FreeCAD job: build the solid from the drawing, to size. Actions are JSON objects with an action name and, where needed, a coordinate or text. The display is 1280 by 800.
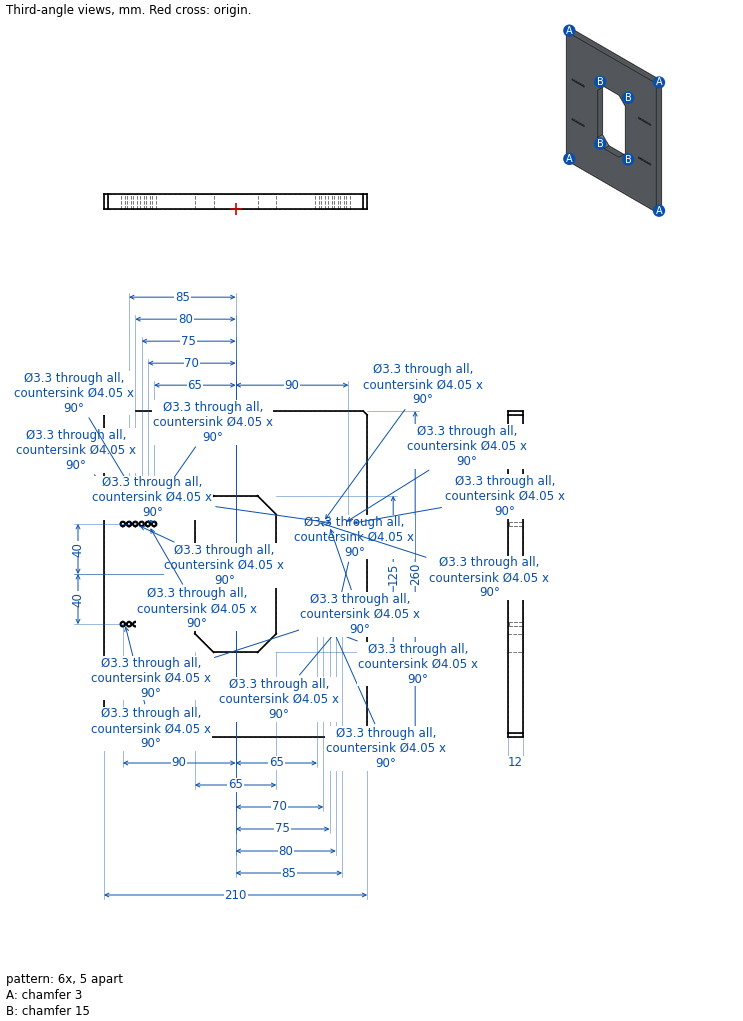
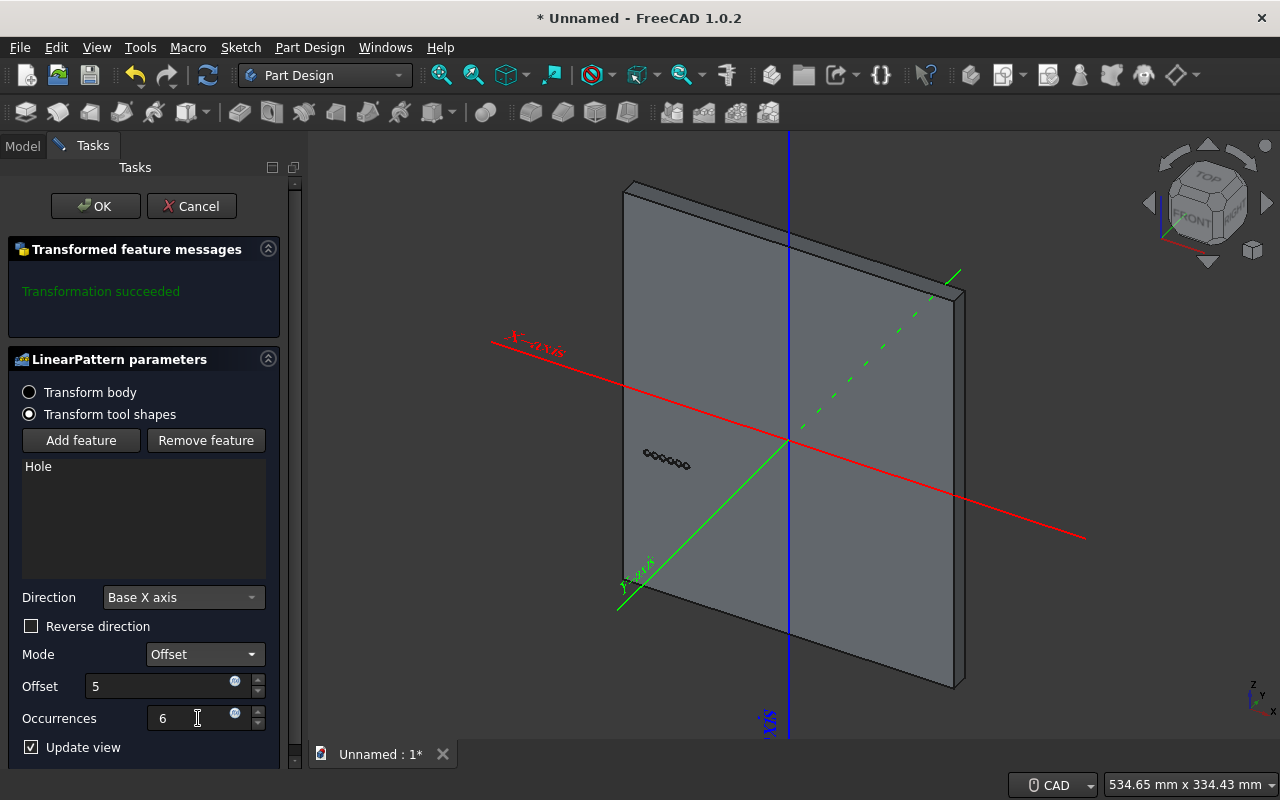
{"action": "left_click", "coordinate": [96, 206]}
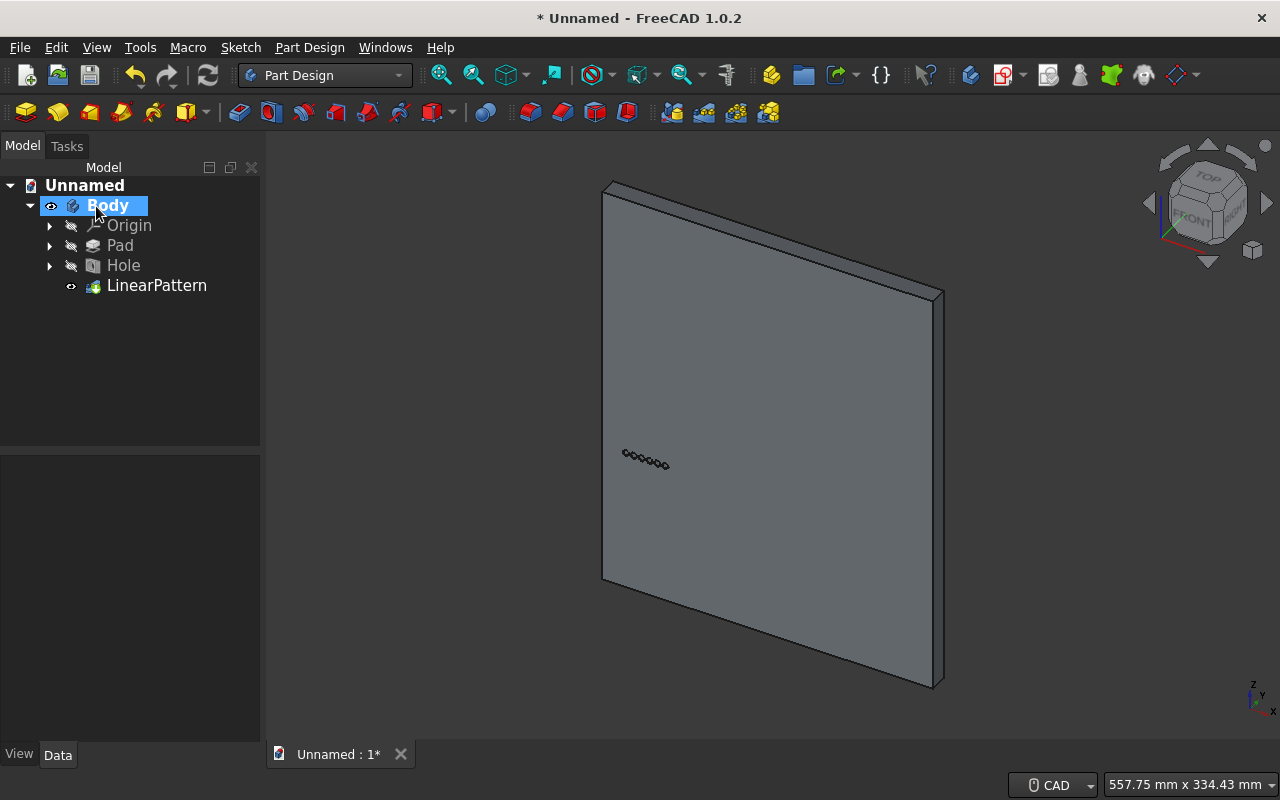
{"action": "left_click", "coordinate": [116, 266]}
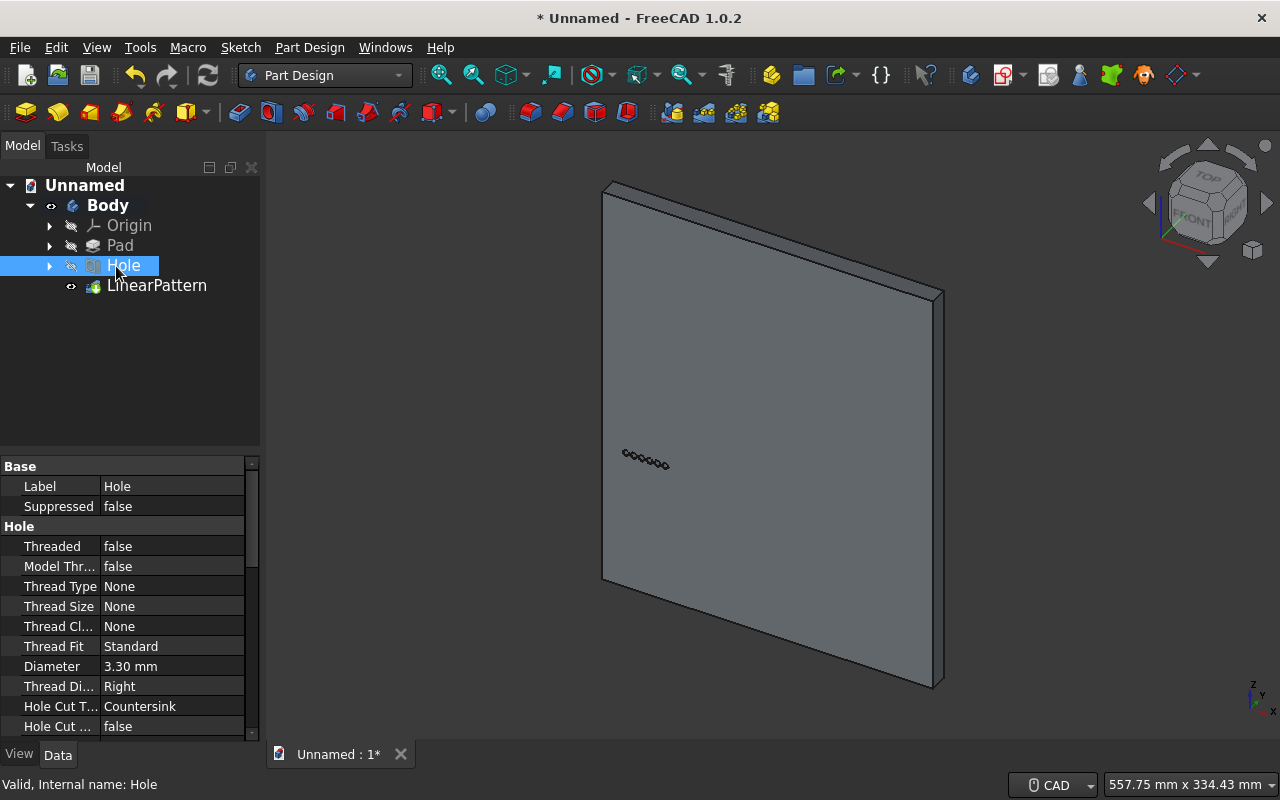
{"action": "left_click", "coordinate": [672, 112]}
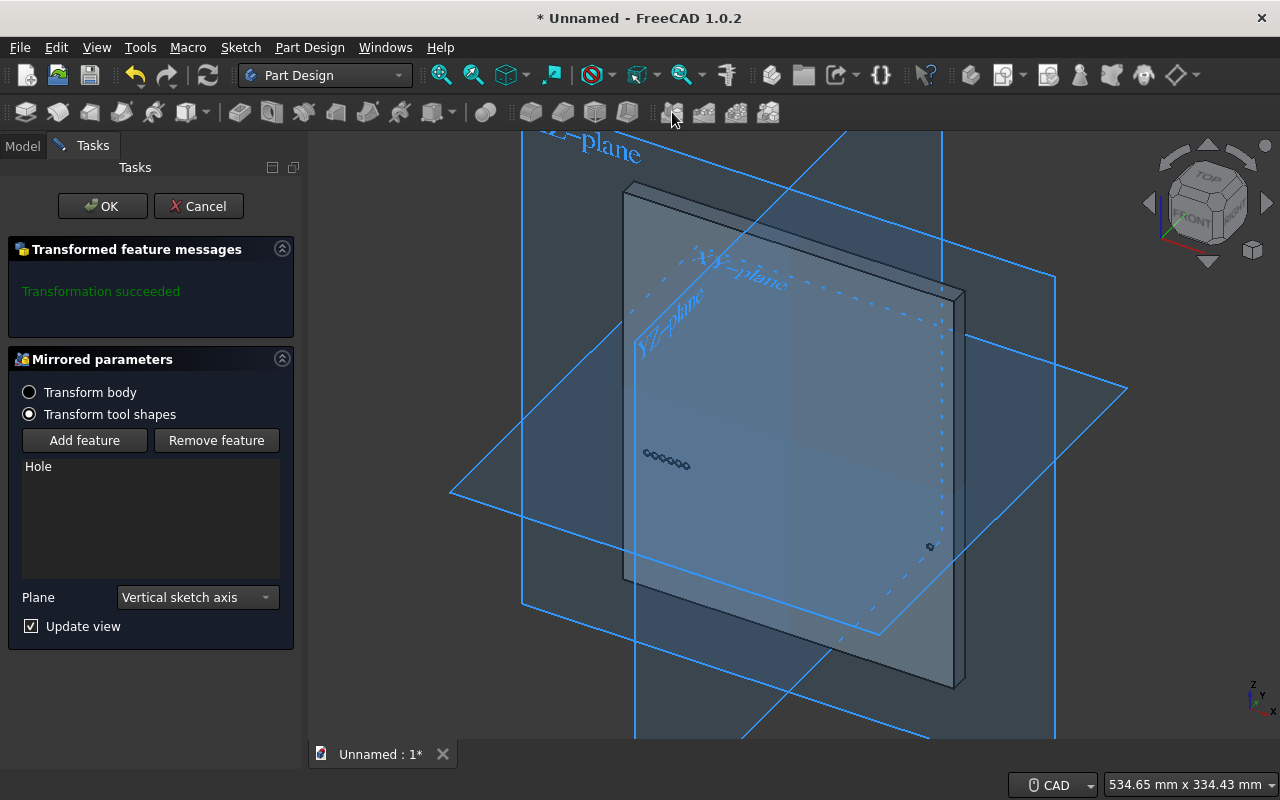
{"action": "left_click", "coordinate": [198, 598]}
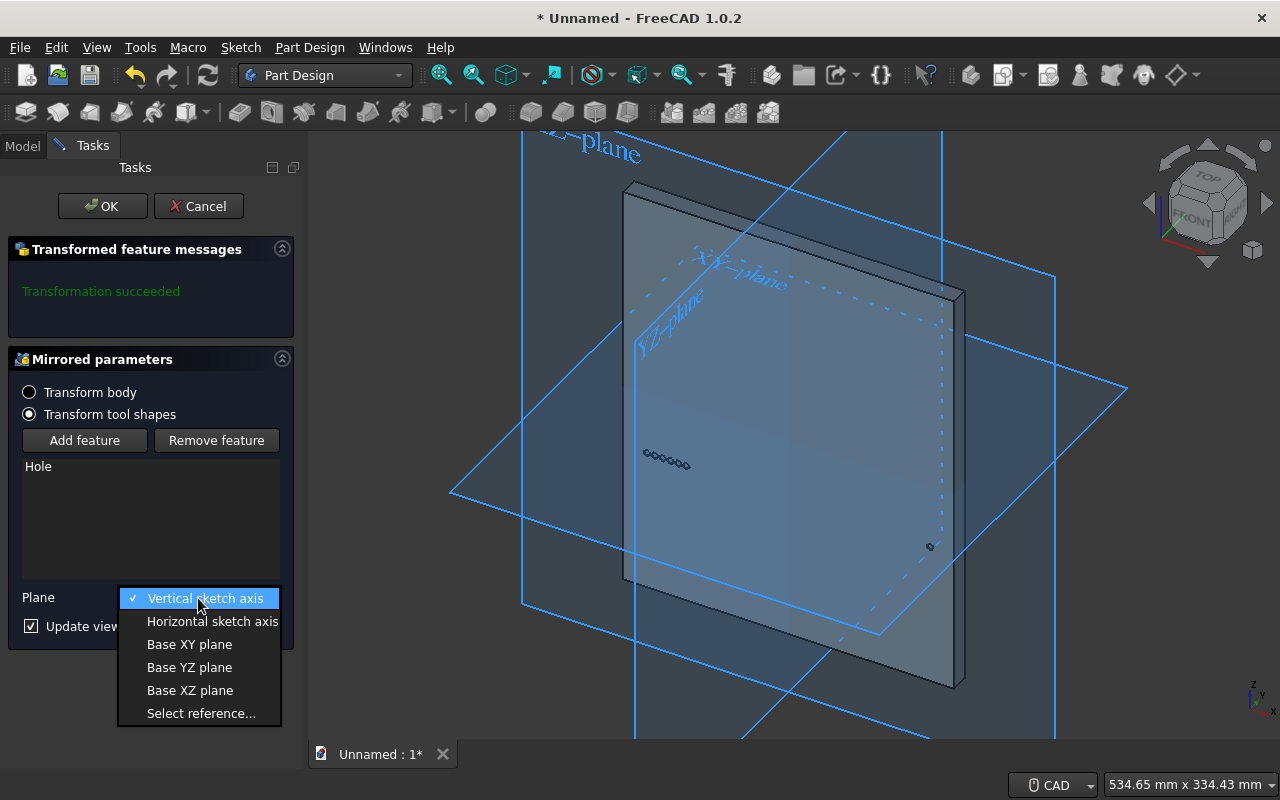
{"action": "left_click", "coordinate": [198, 668]}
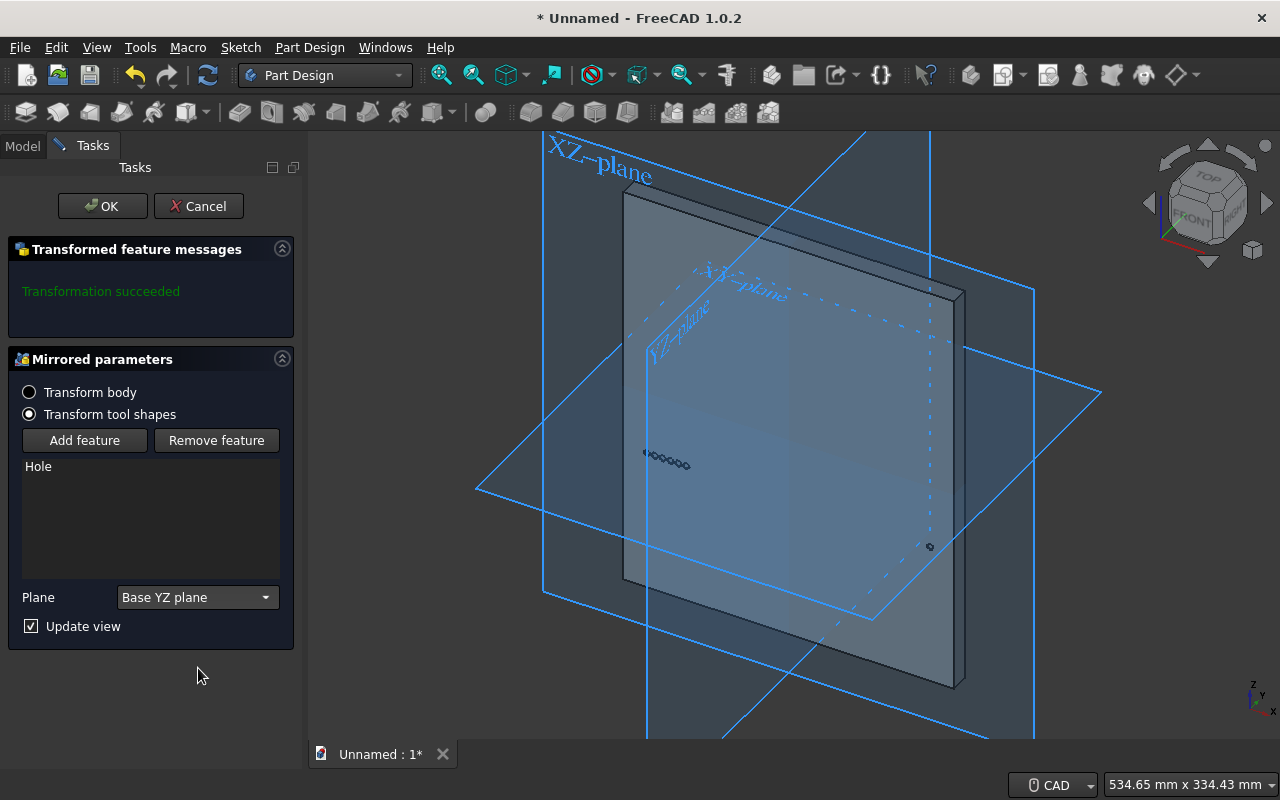
{"action": "left_click", "coordinate": [103, 206]}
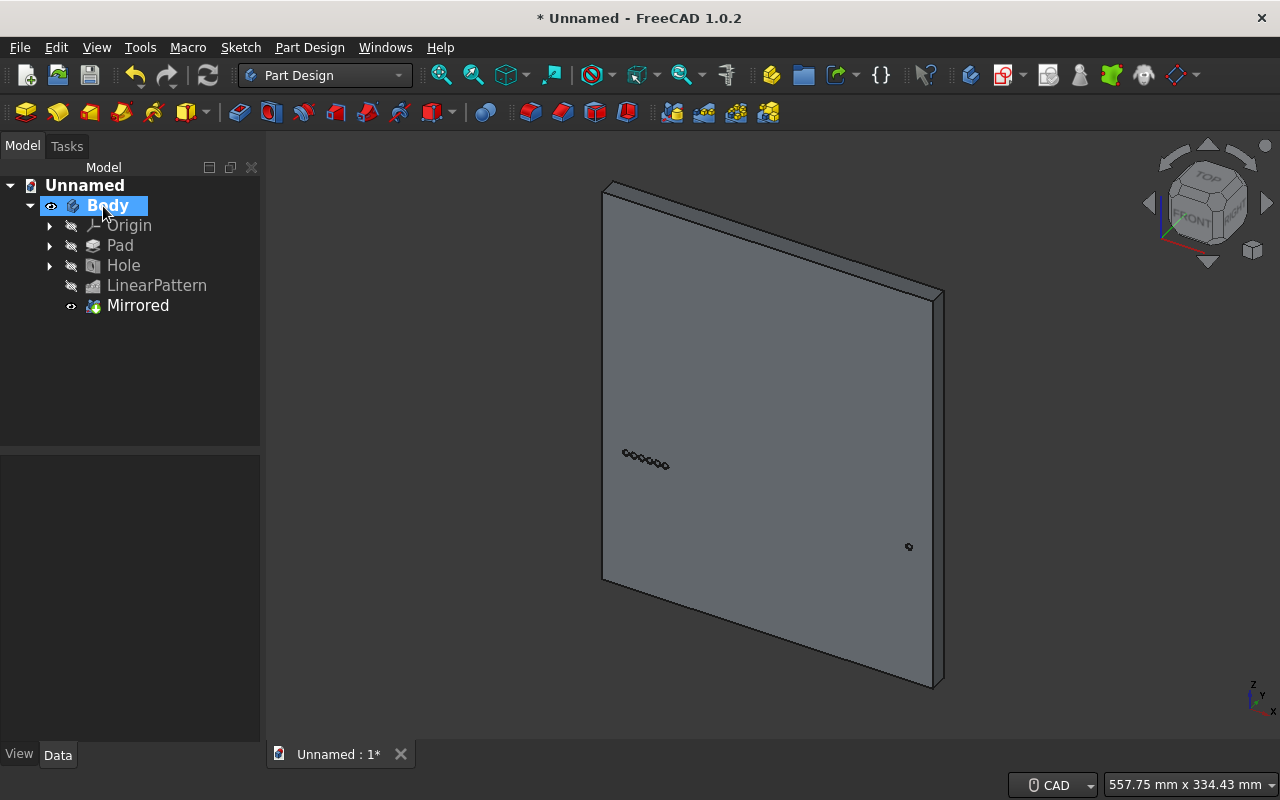
{"action": "left_click", "coordinate": [768, 384]}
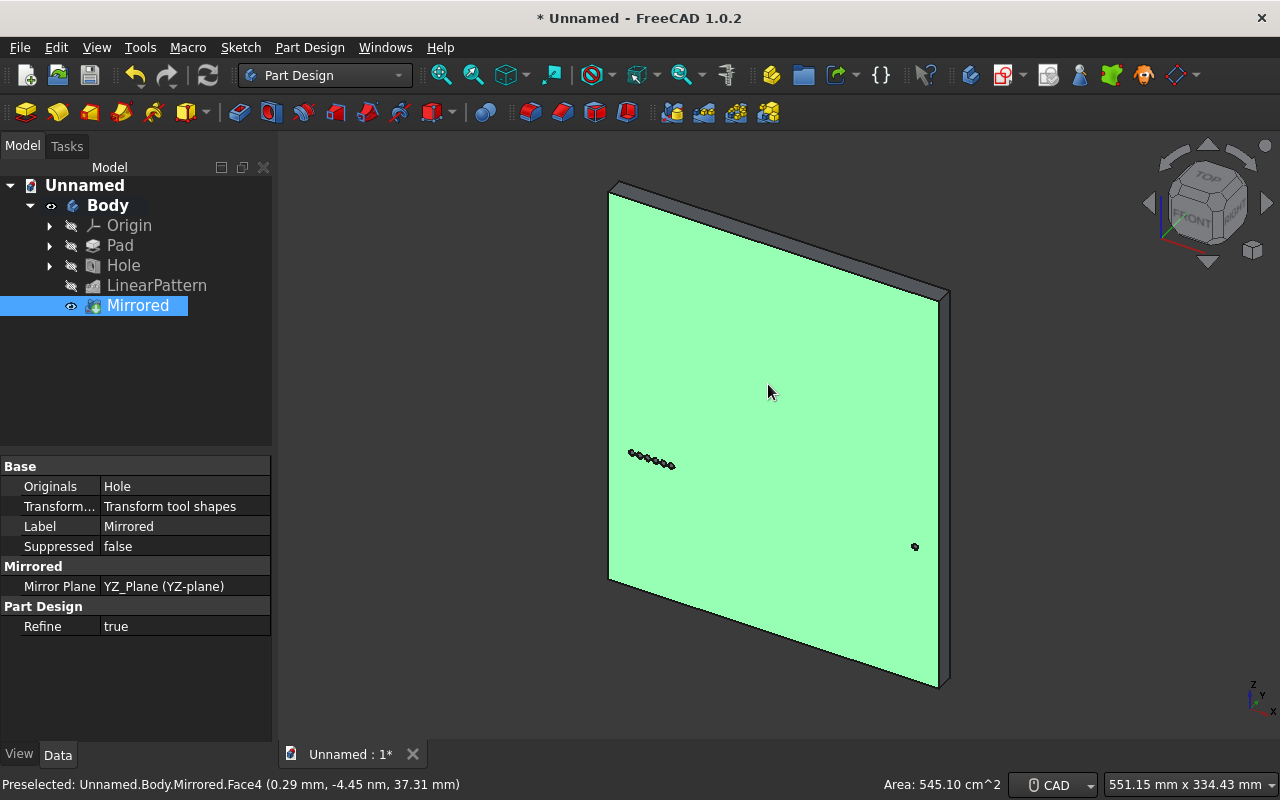
{"action": "left_click", "coordinate": [1004, 76]}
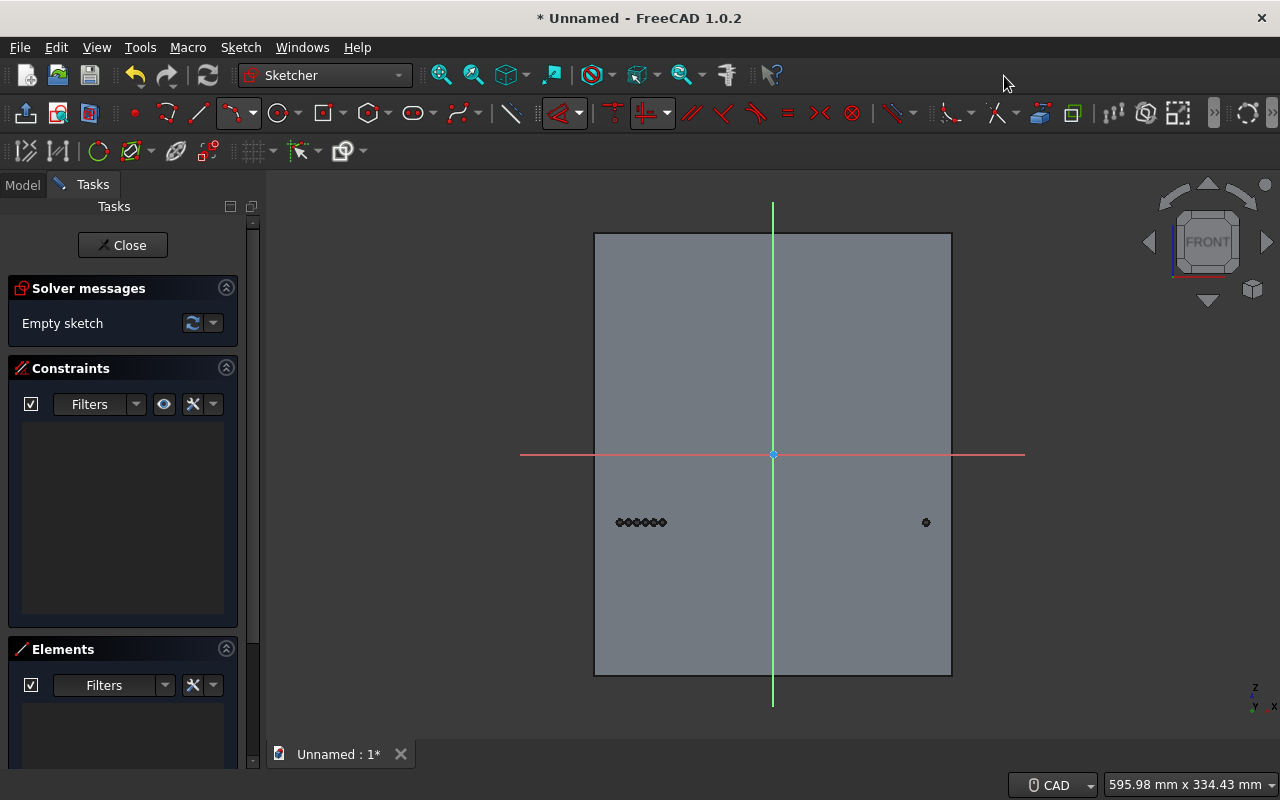
{"action": "scroll", "coordinate": [929, 526], "scroll_direction": "up", "scroll_amount": 15}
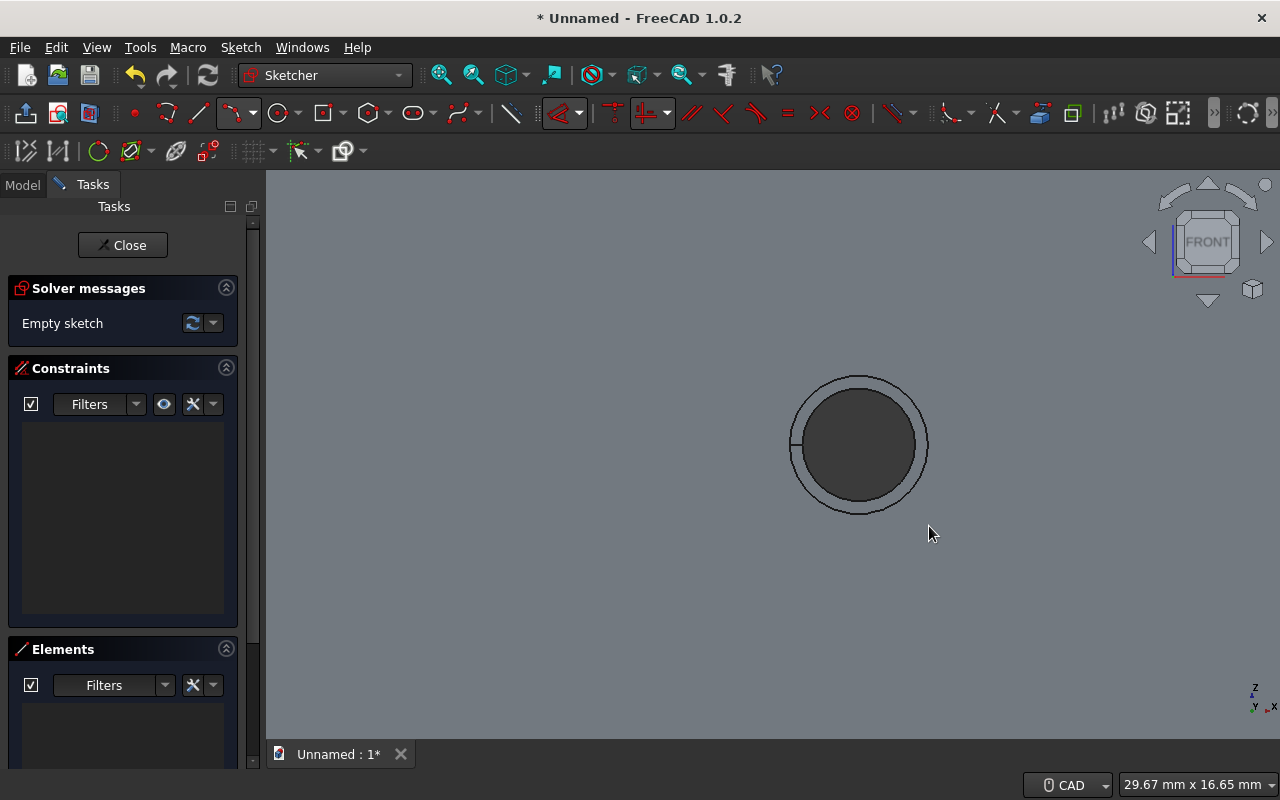
{"action": "scroll", "coordinate": [681, 441], "scroll_direction": "up", "scroll_amount": 6}